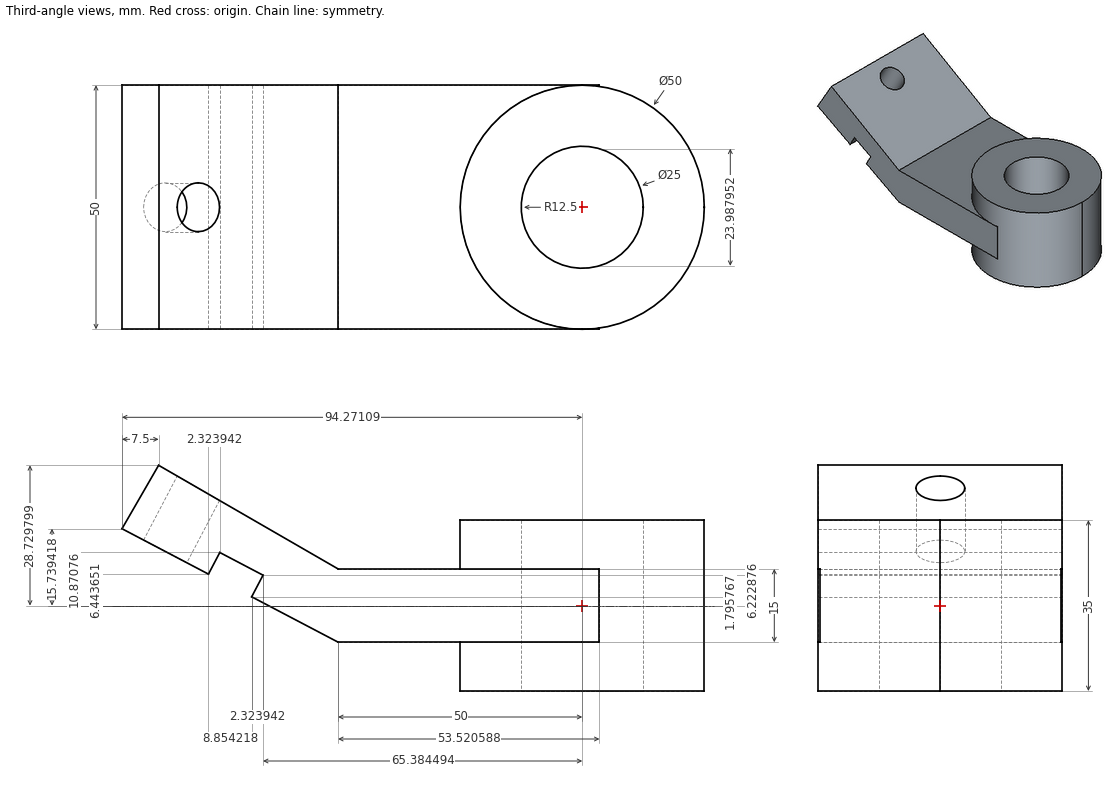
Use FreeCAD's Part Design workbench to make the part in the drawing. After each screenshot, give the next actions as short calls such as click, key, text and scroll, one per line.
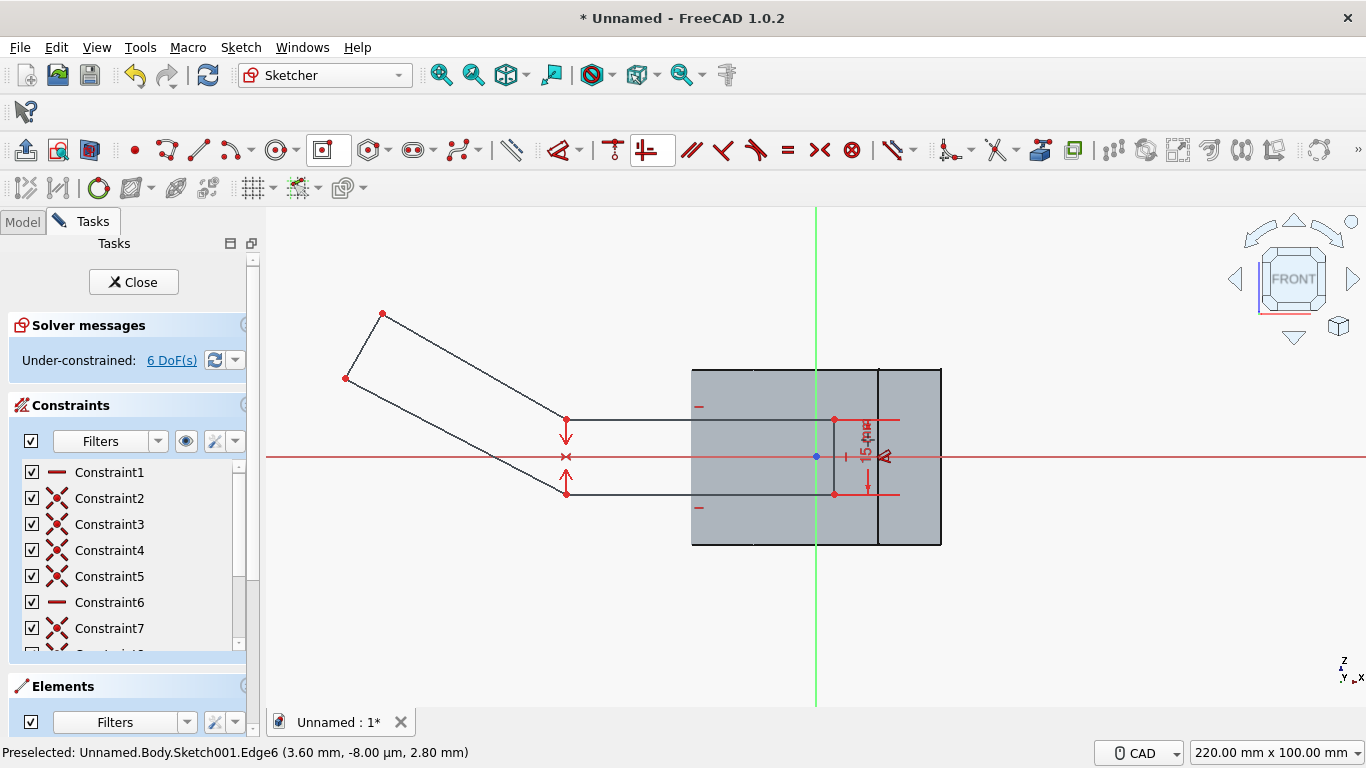
click(566, 494)
click(691, 528)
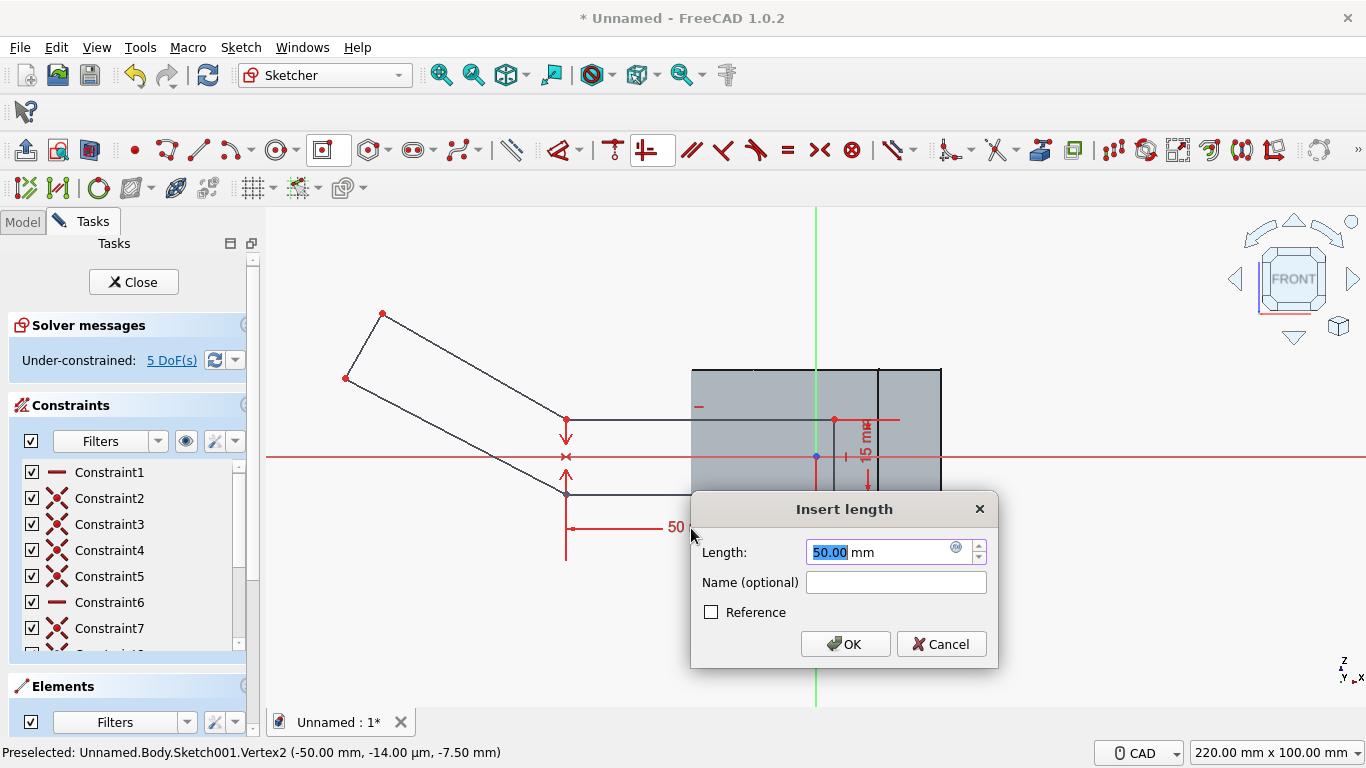
text(50)
key(Return)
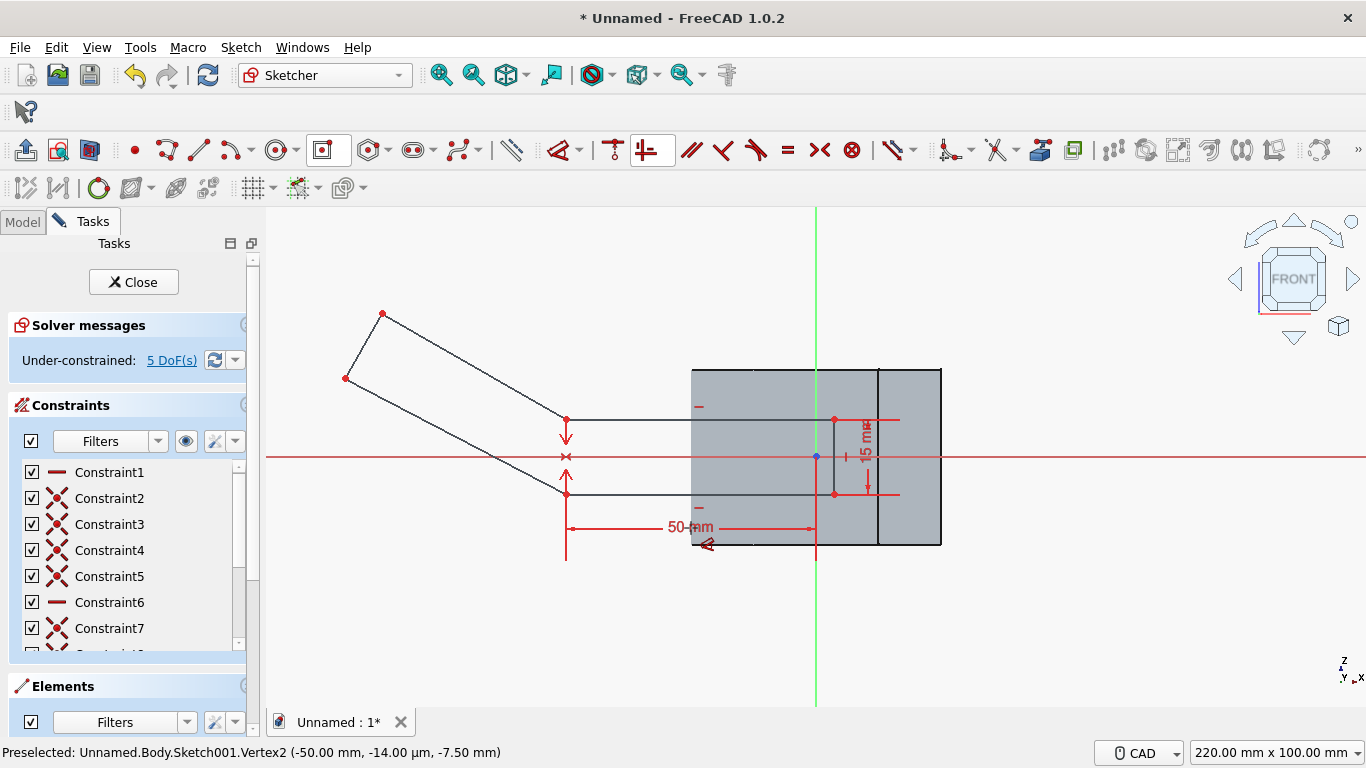
click(356, 359)
click(363, 280)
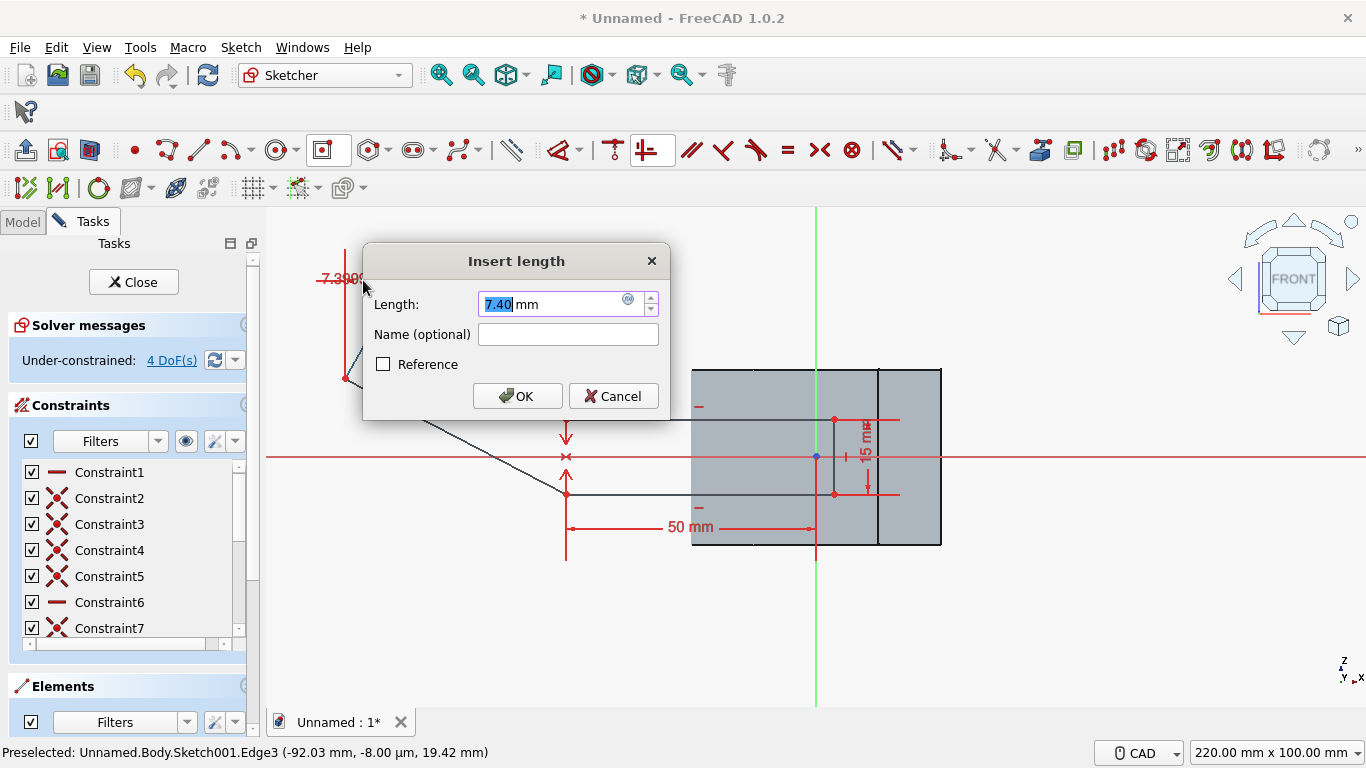
text(7.5)
key(Return)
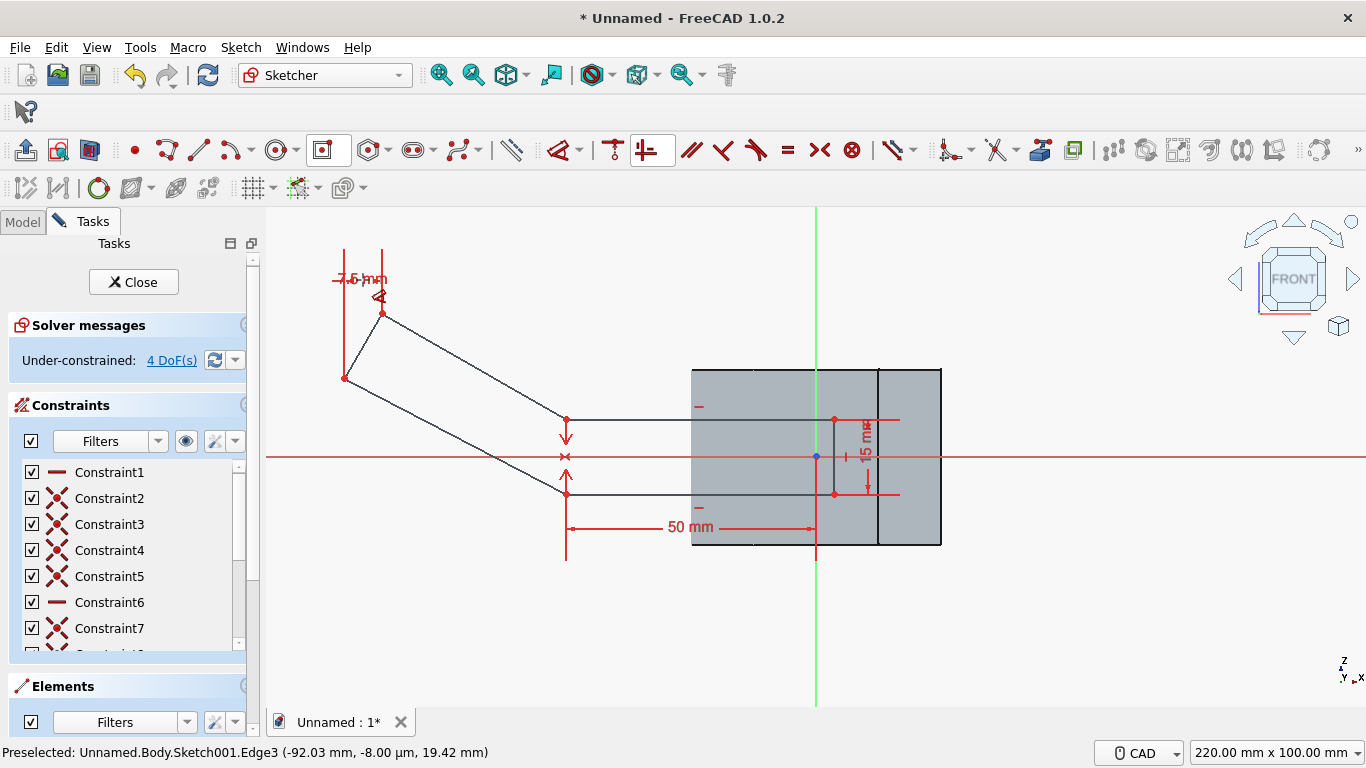
click(754, 494)
click(762, 528)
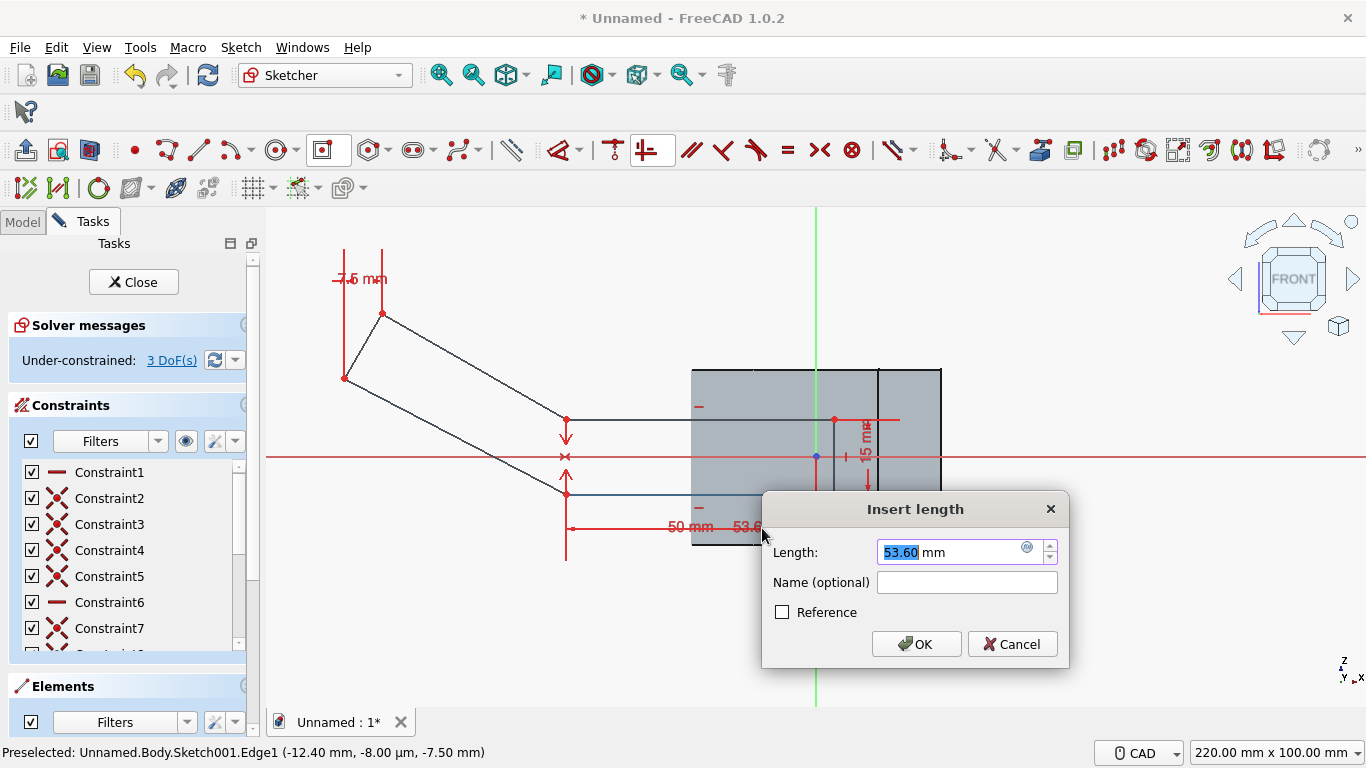
text(53.520588)
key(Return)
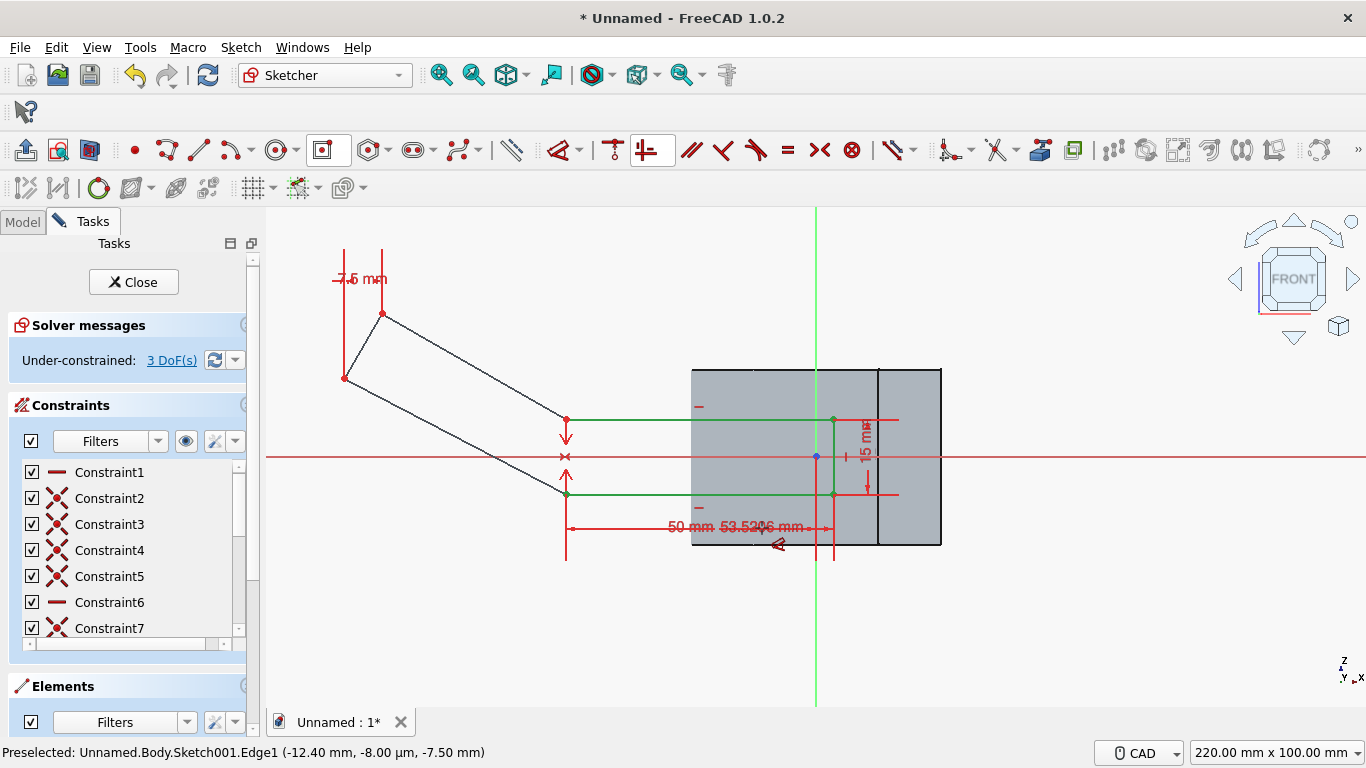
click(344, 379)
click(472, 491)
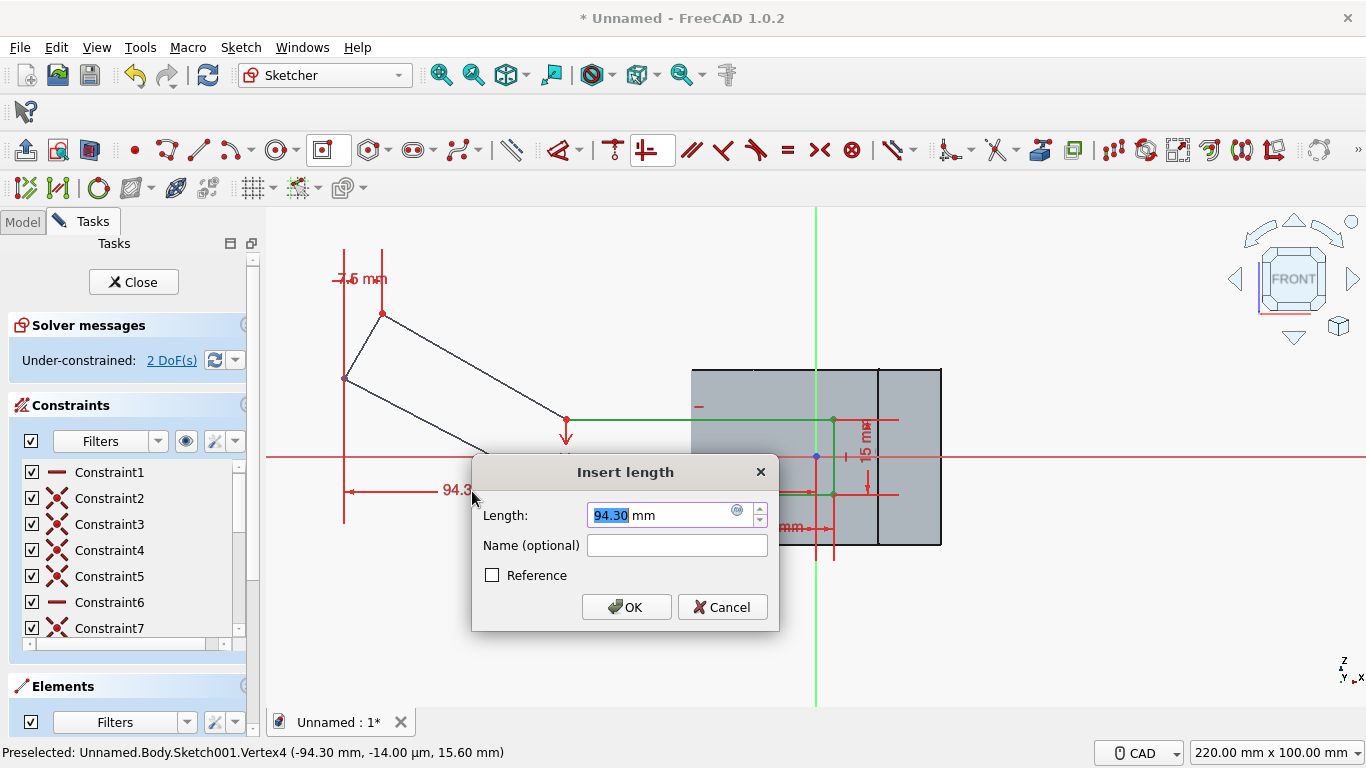
text(94.27109)
key(Return)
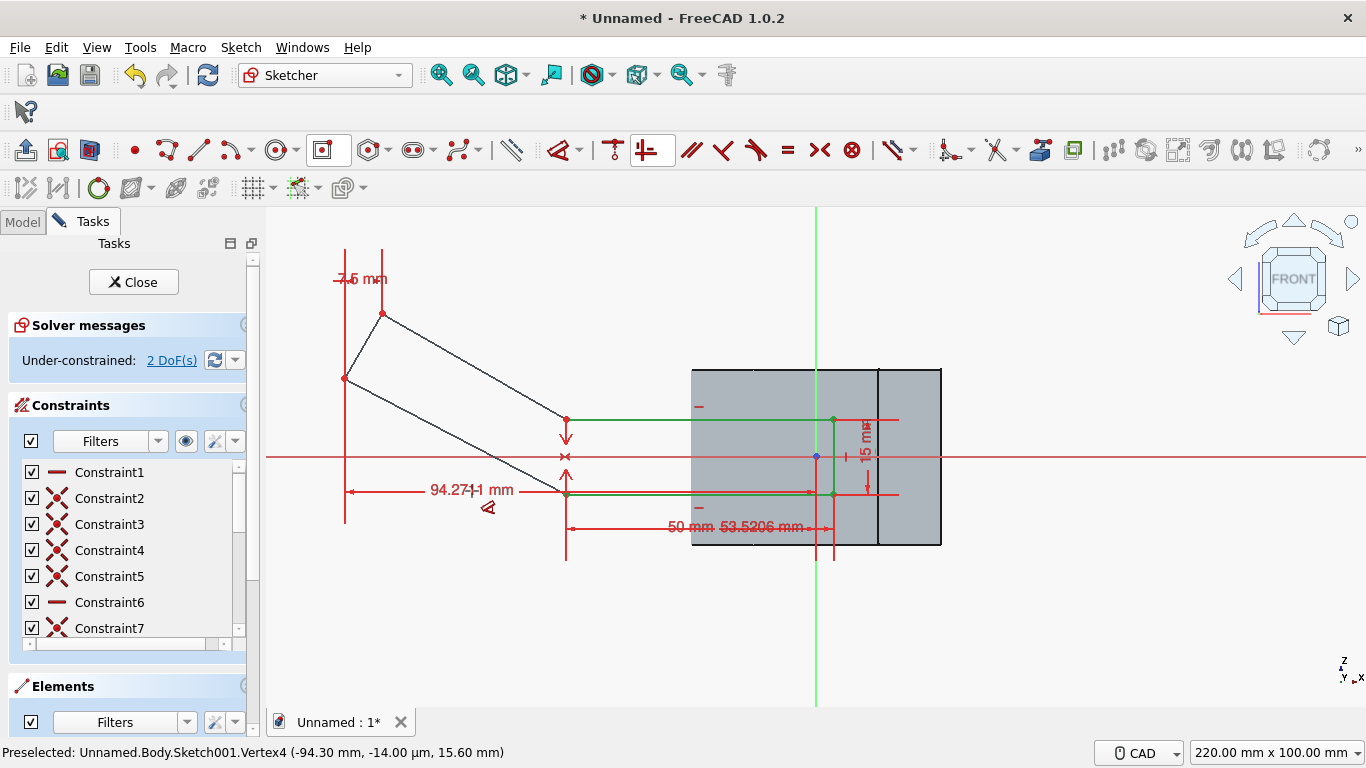
click(345, 379)
click(311, 418)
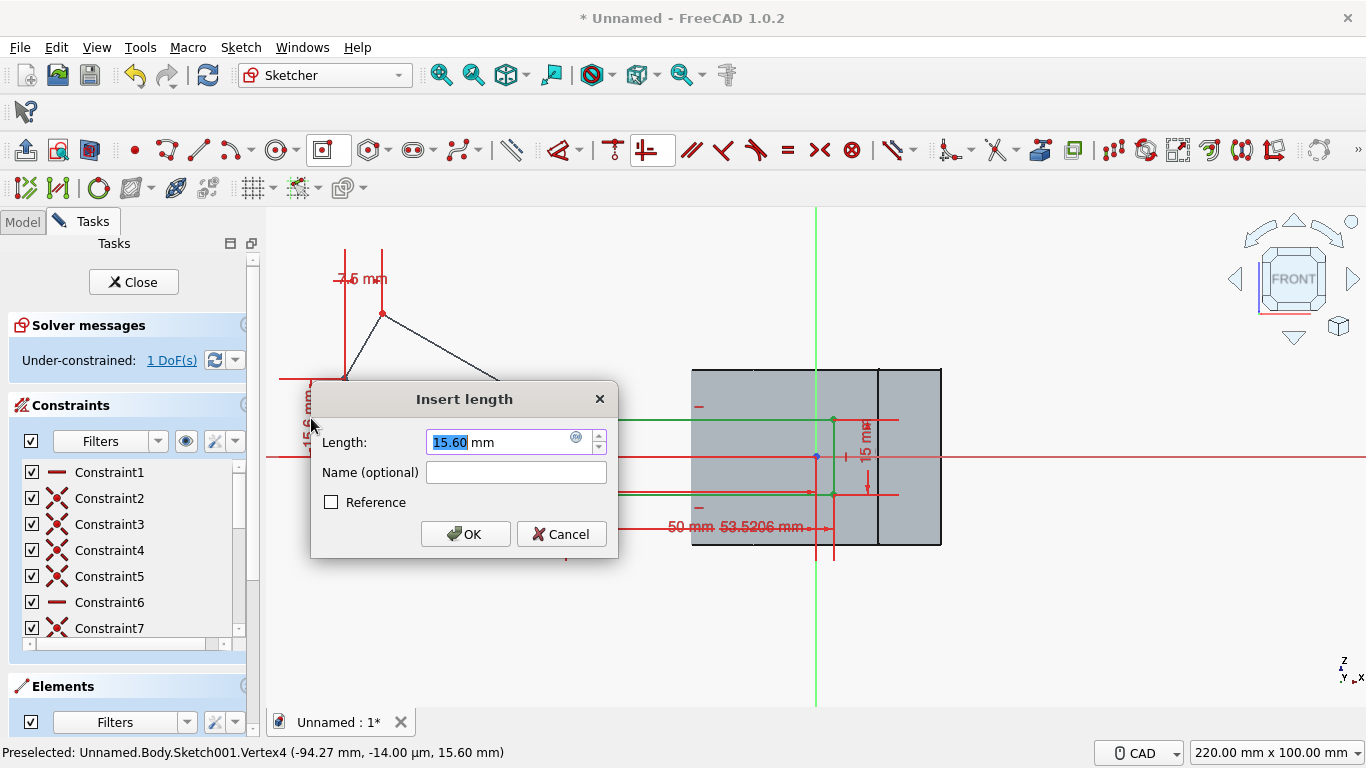
text(15.739418)
key(Return)